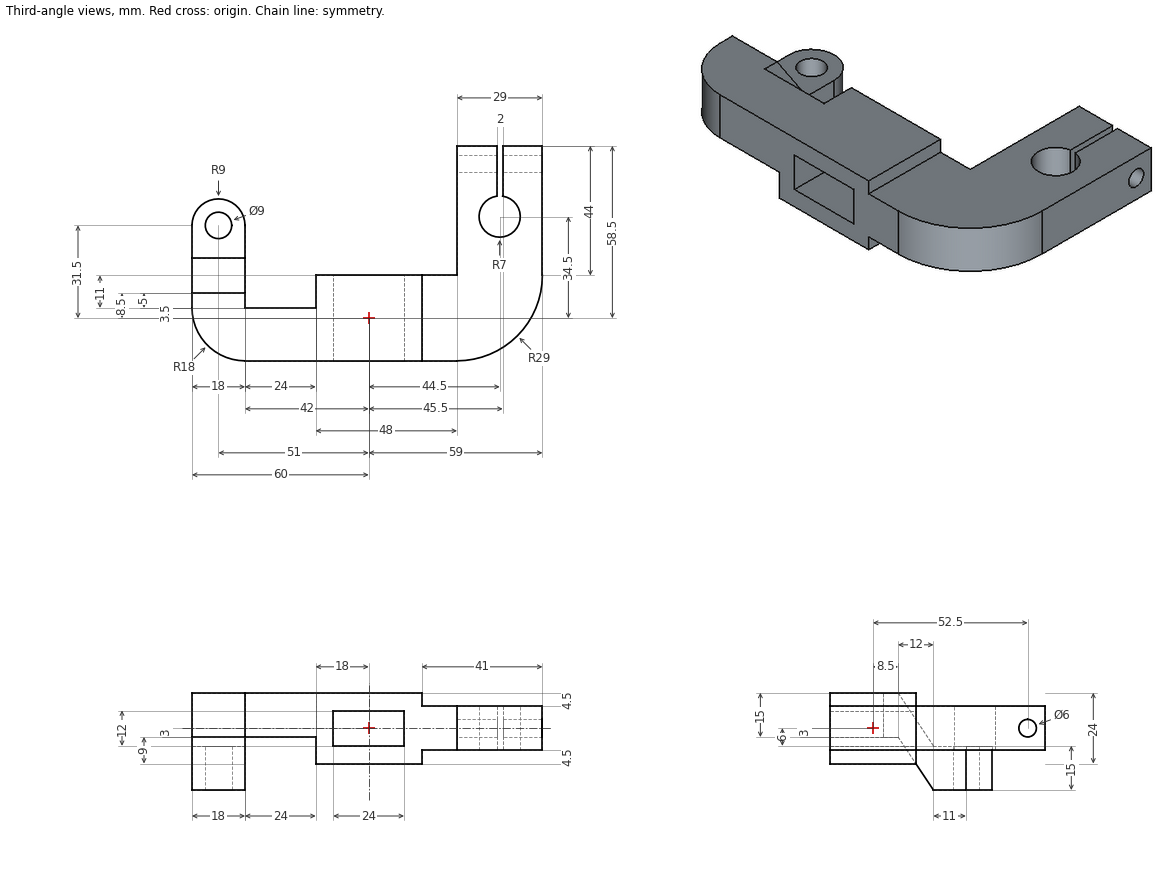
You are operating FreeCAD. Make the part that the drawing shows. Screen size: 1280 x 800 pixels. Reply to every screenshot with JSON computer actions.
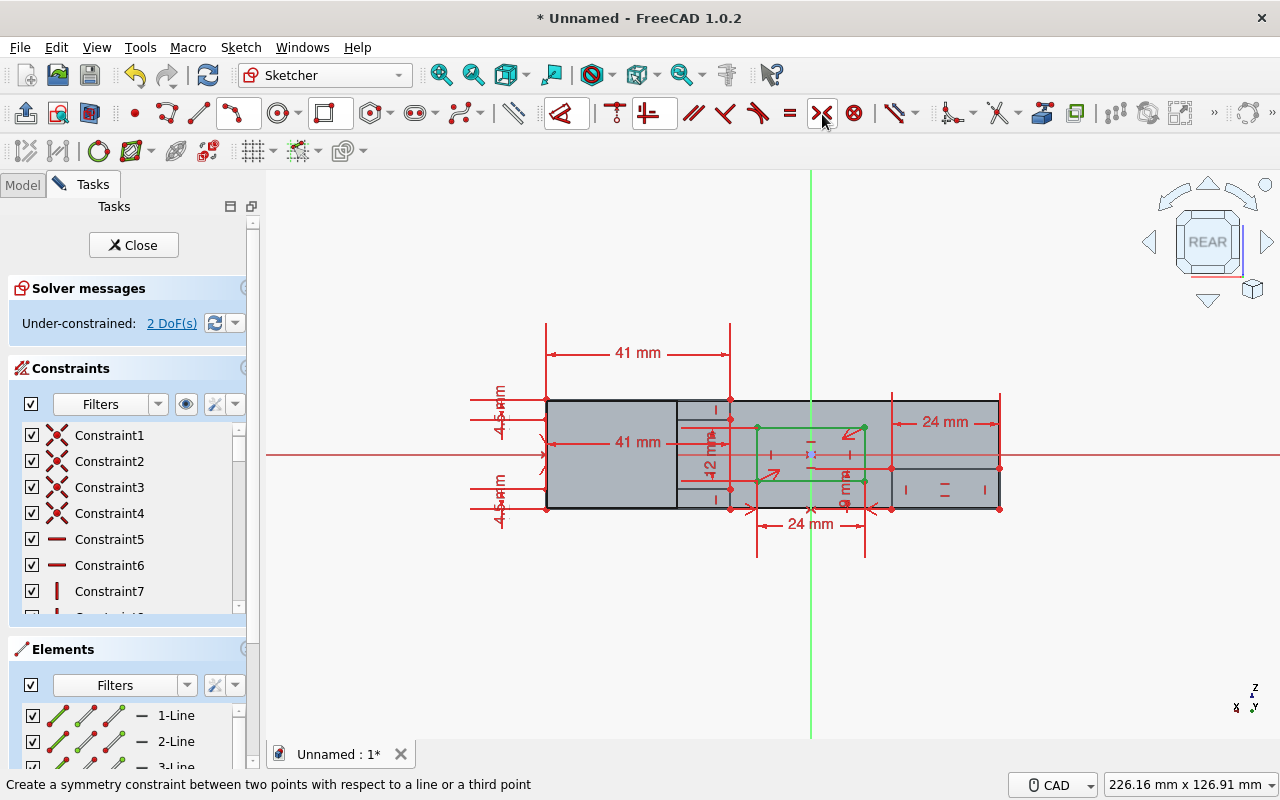
{"action": "scroll", "coordinate": [892, 469], "scroll_direction": "up", "scroll_amount": 6}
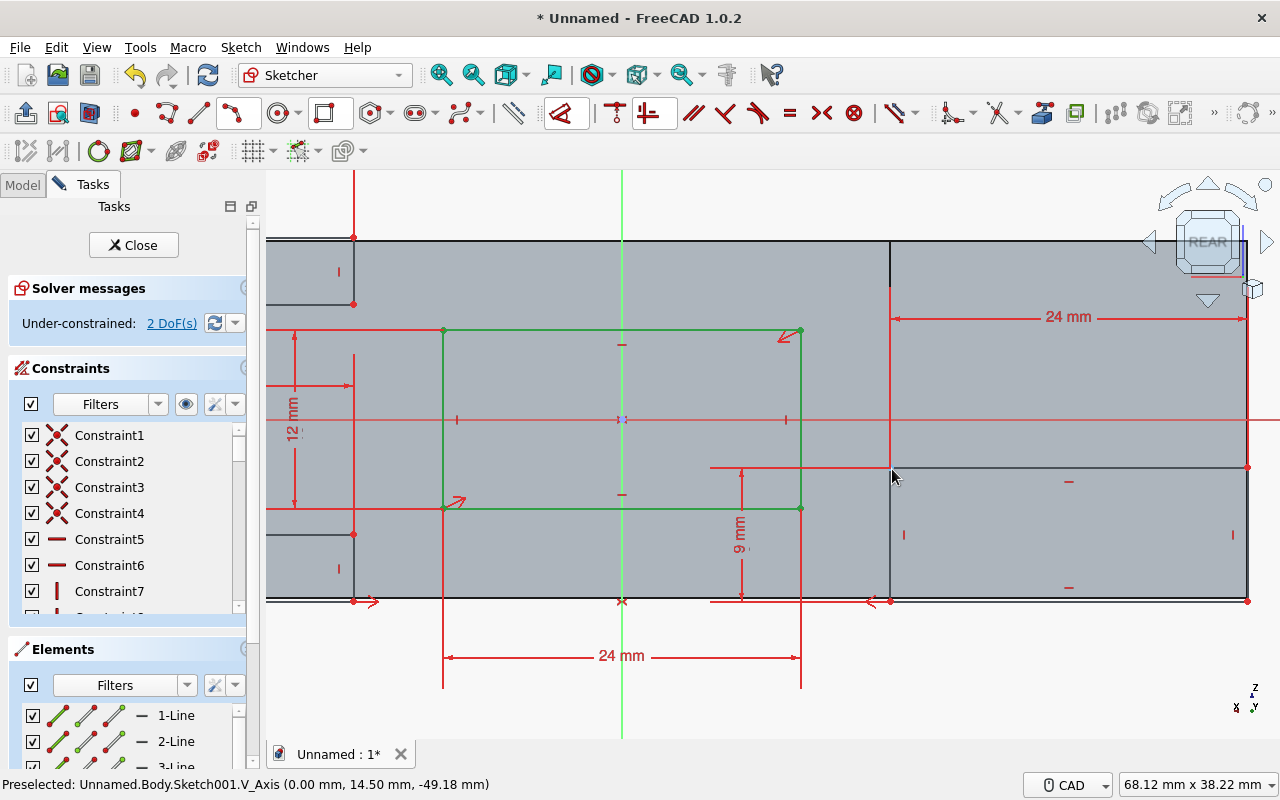
{"action": "left_click", "coordinate": [890, 468]}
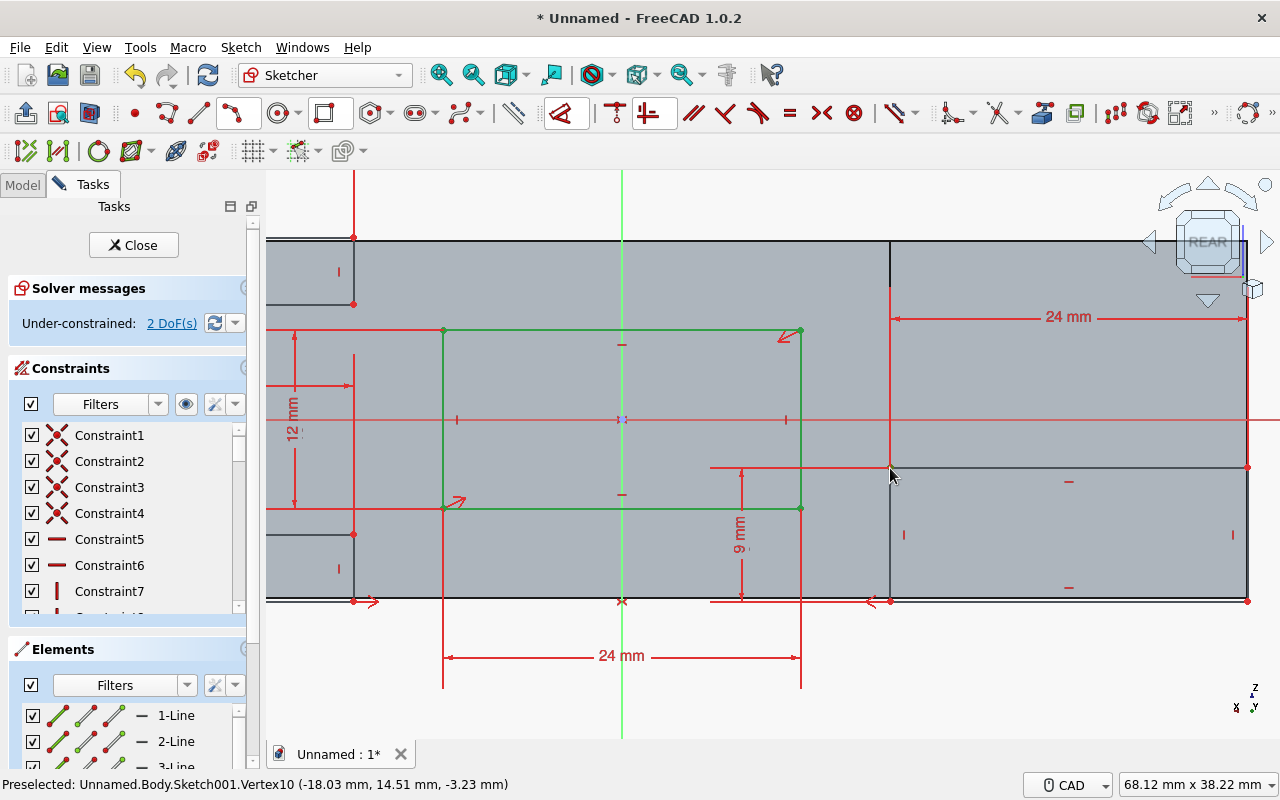
{"action": "left_click", "coordinate": [584, 114]}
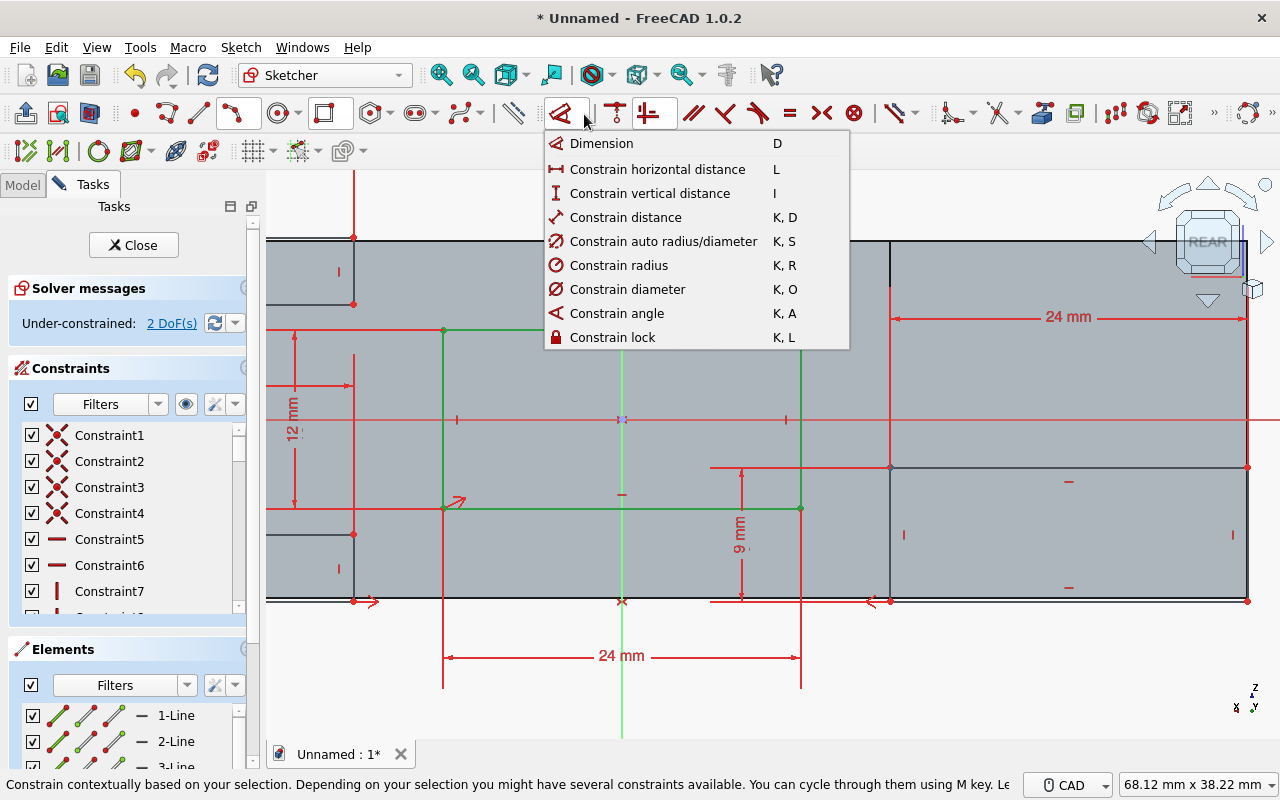
{"action": "left_click", "coordinate": [697, 193]}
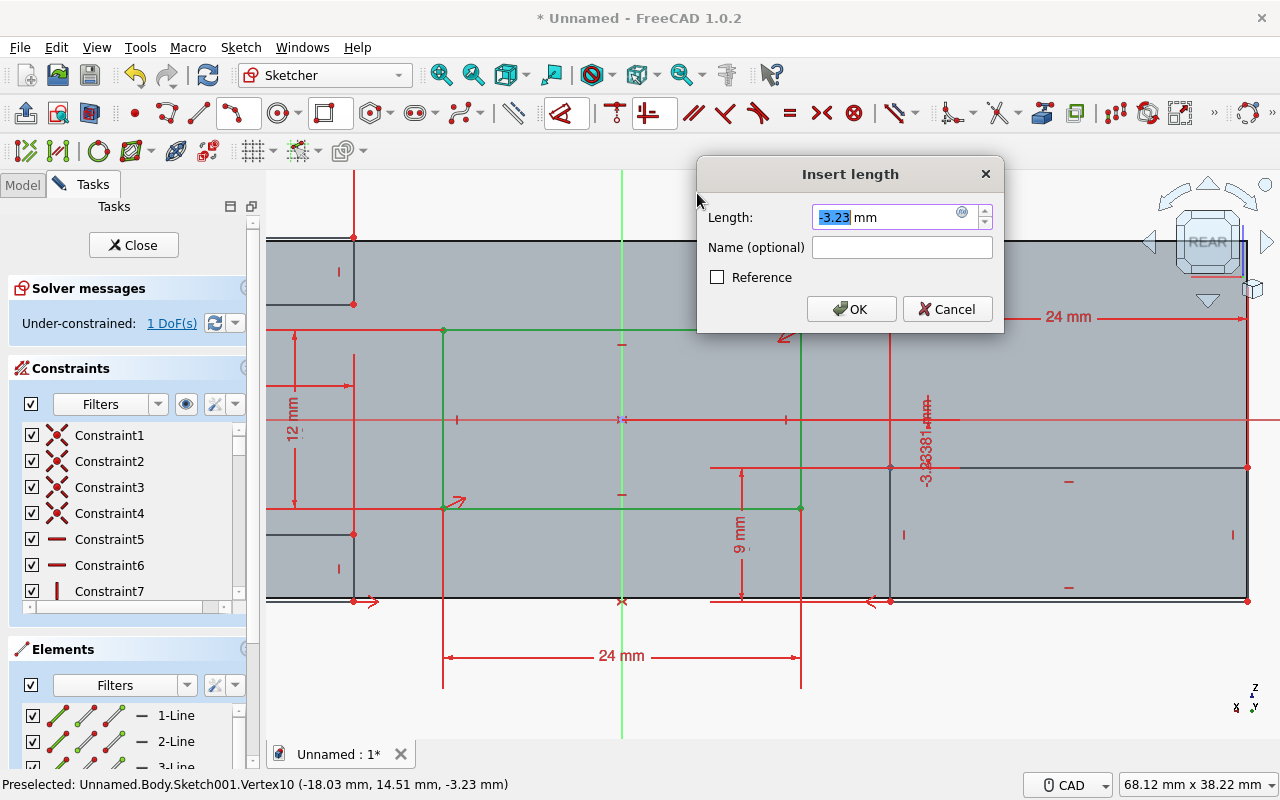
{"action": "type", "text": "-3"}
{"action": "key", "text": "Return"}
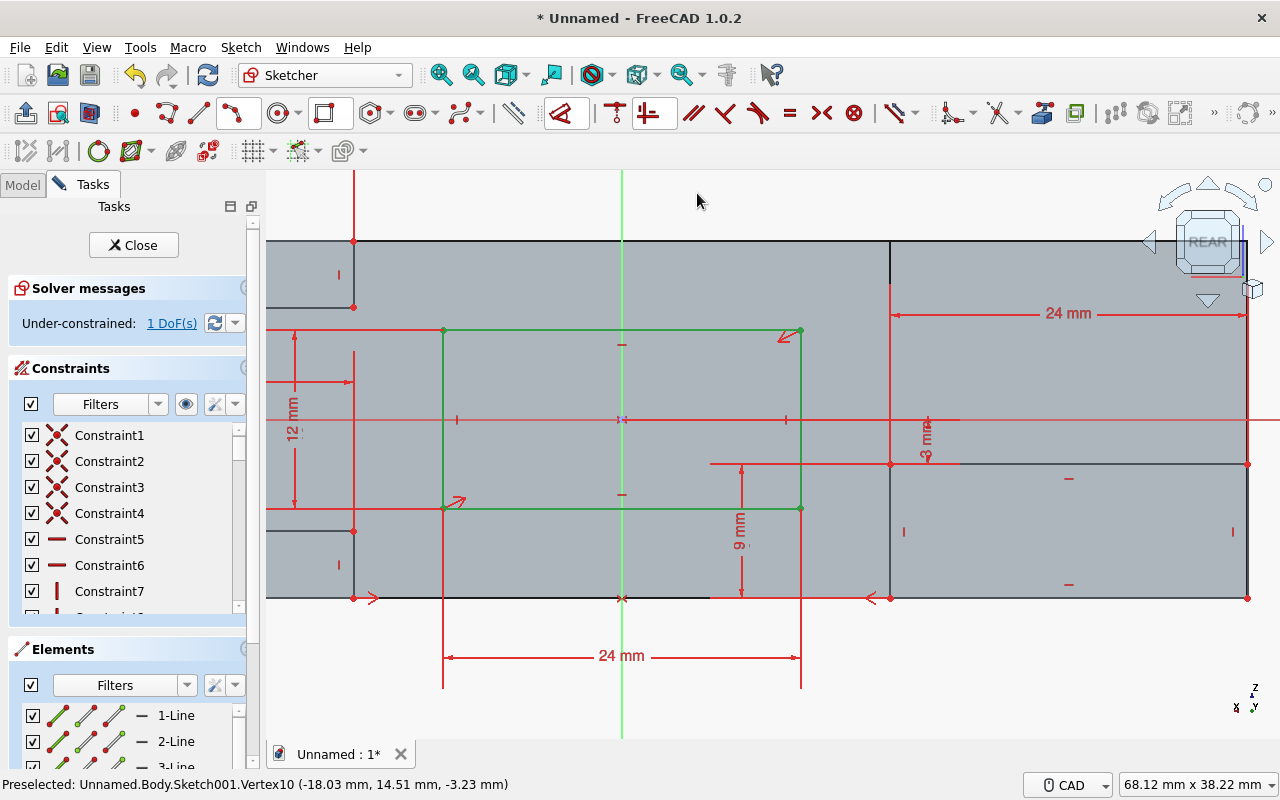
{"action": "left_click", "coordinate": [890, 464]}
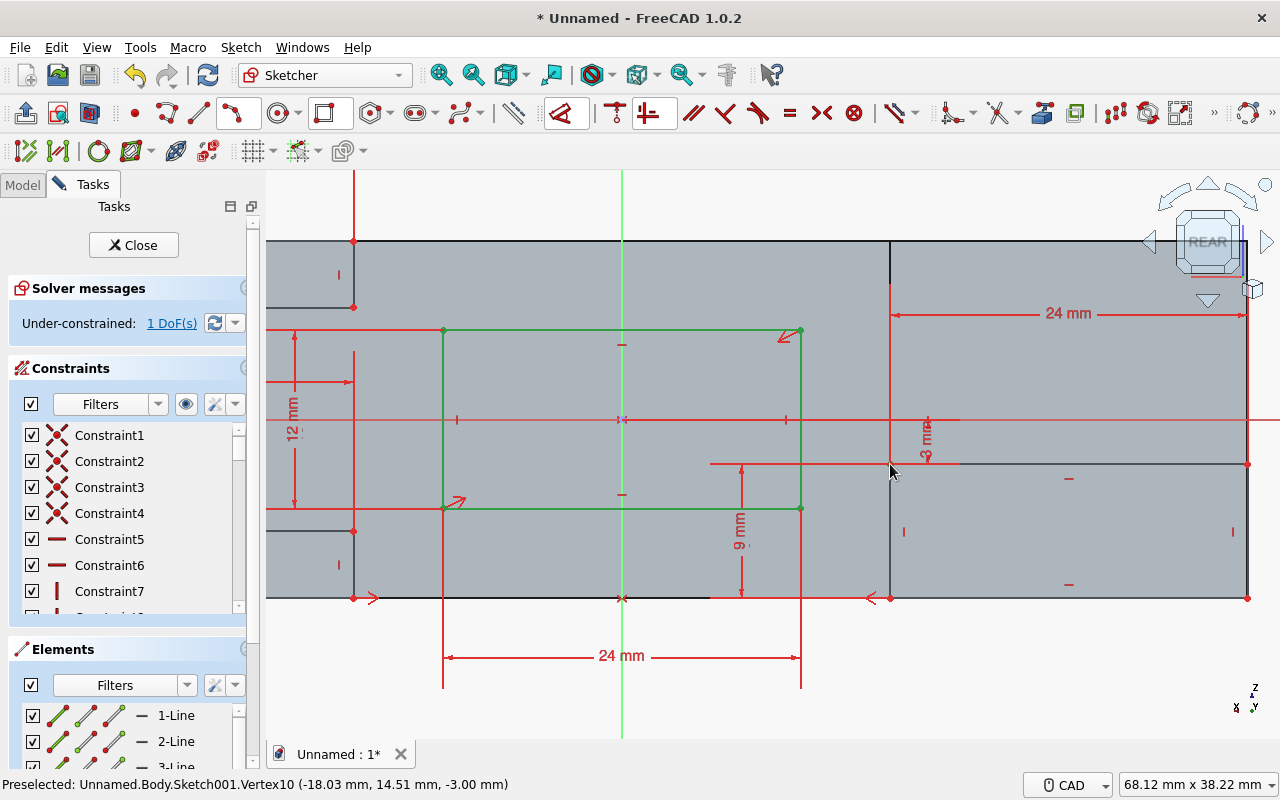
{"action": "key", "text": "l"}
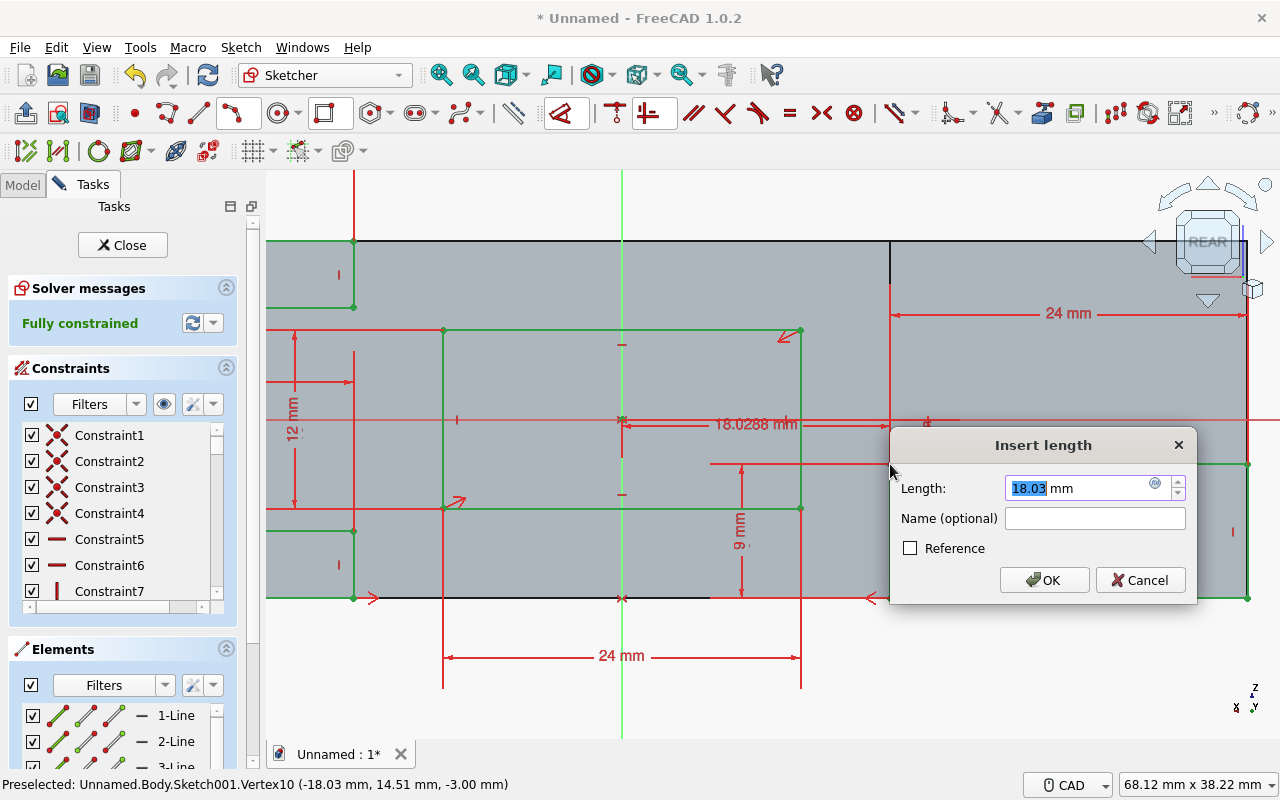
{"action": "type", "text": "18"}
{"action": "key", "text": "Return"}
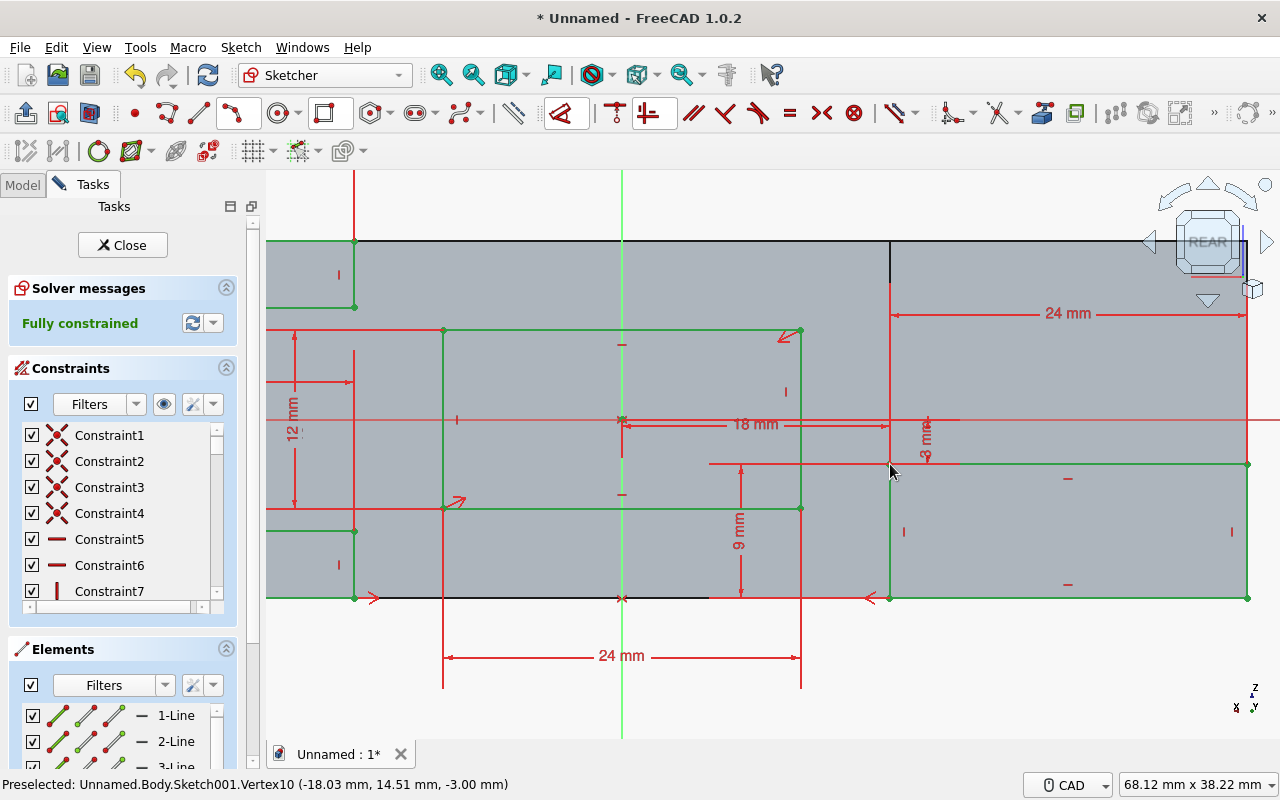
{"action": "left_click", "coordinate": [123, 245]}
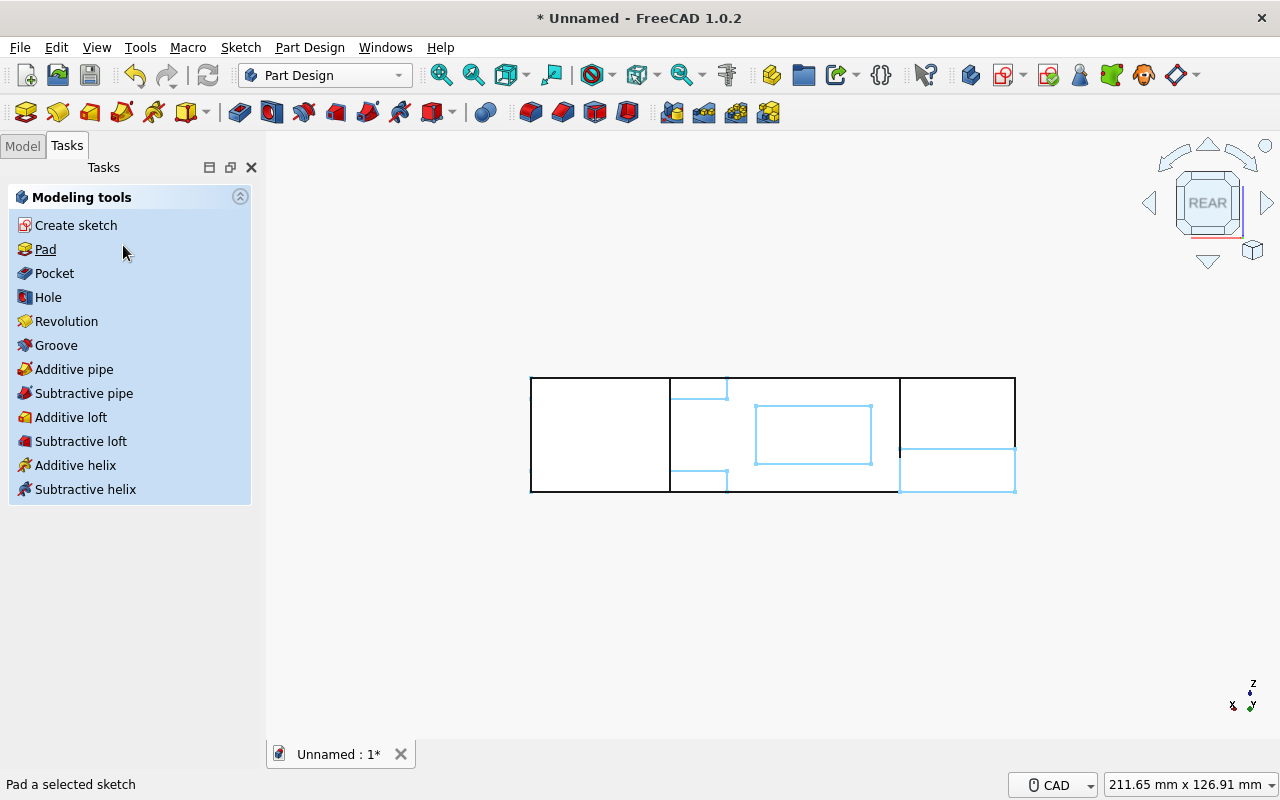
{"action": "left_click", "coordinate": [240, 112]}